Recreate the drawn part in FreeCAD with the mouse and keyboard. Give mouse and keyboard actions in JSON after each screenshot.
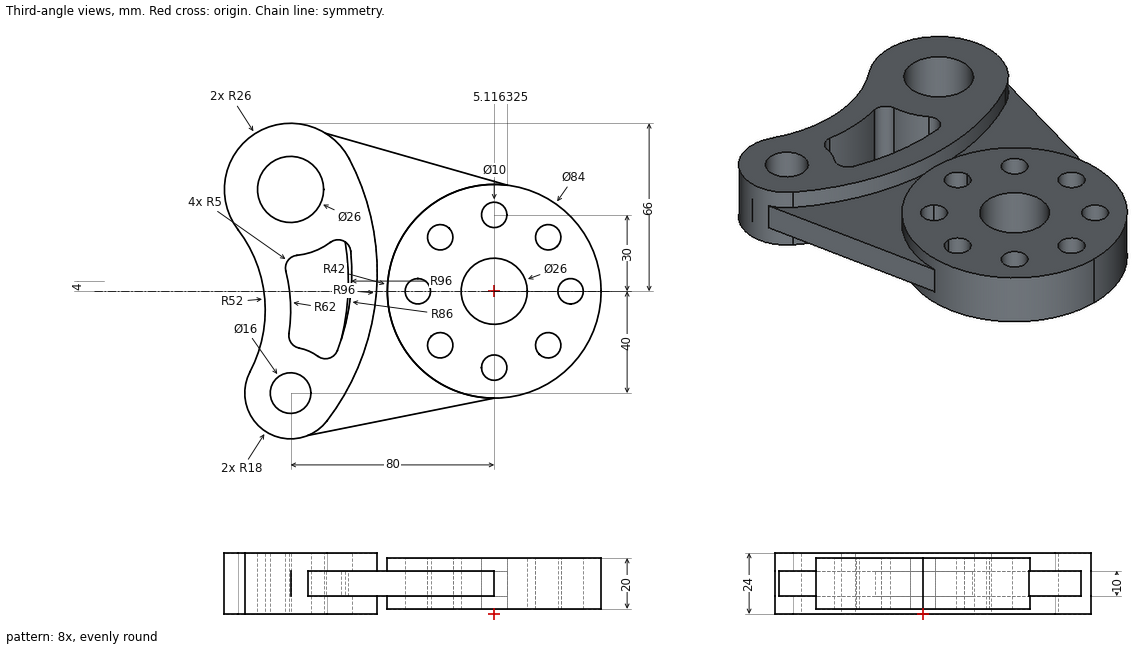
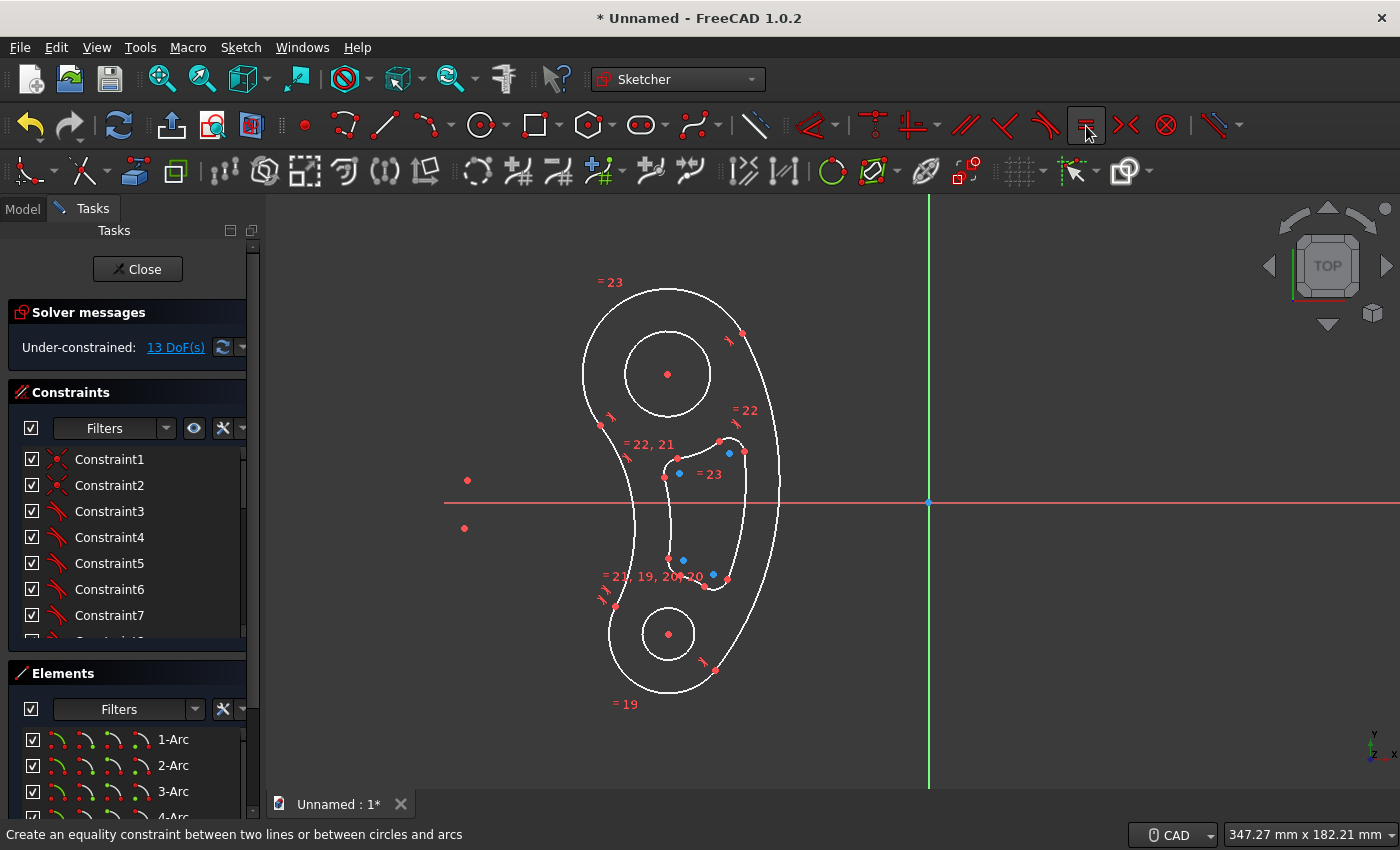
{"action": "left_click", "coordinate": [668, 374]}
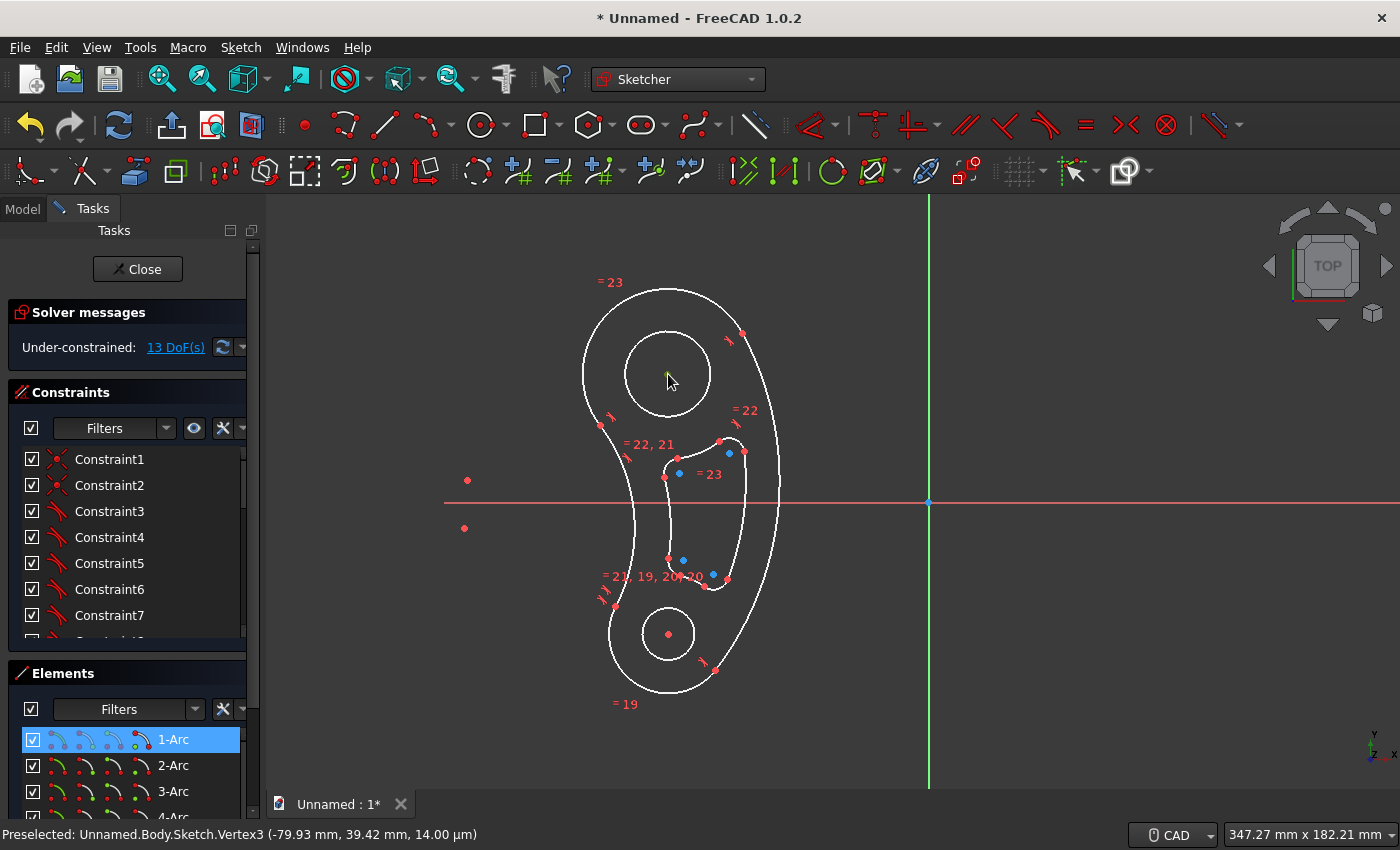
{"action": "left_click", "coordinate": [668, 634]}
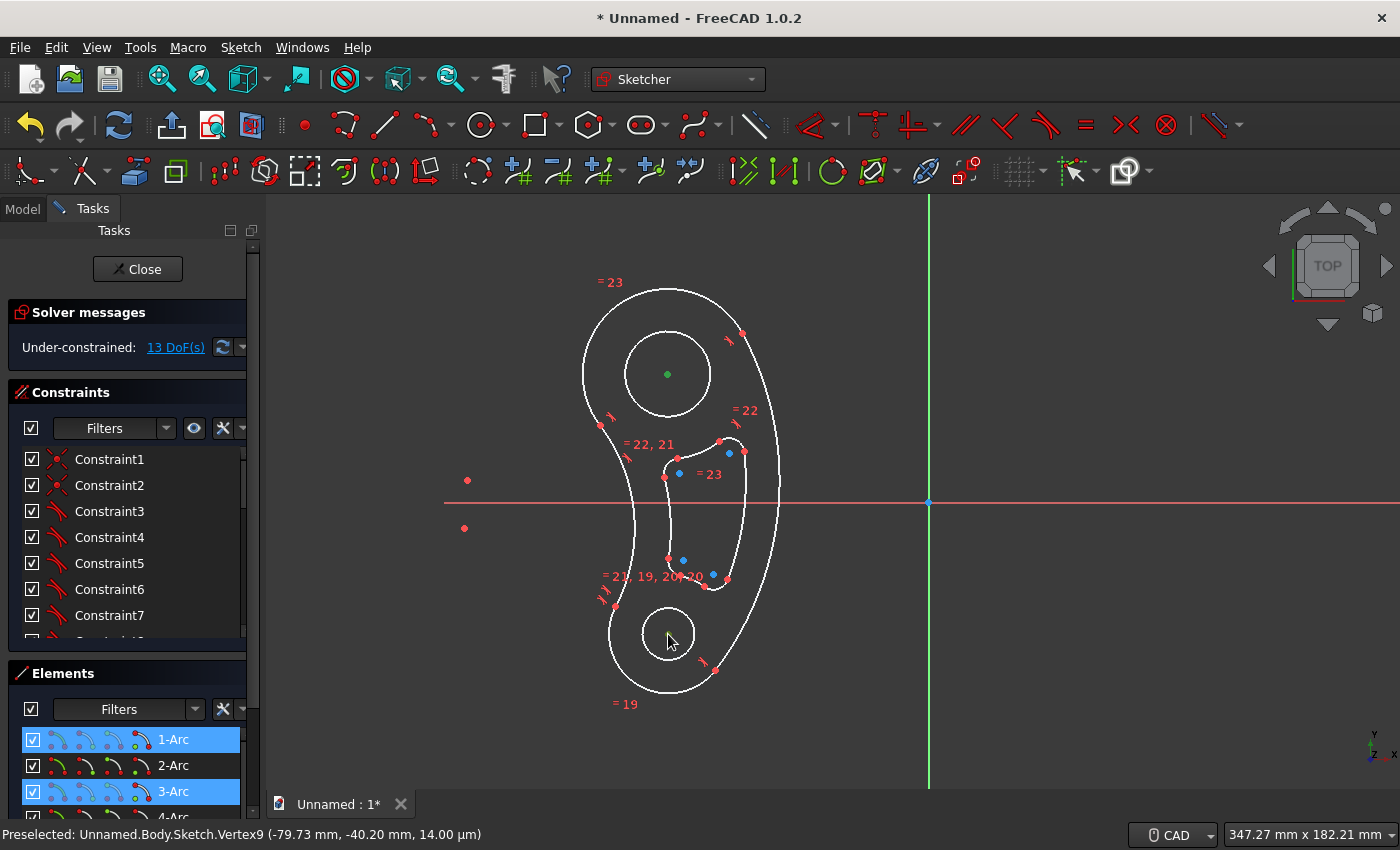
{"action": "left_click", "coordinate": [496, 503]}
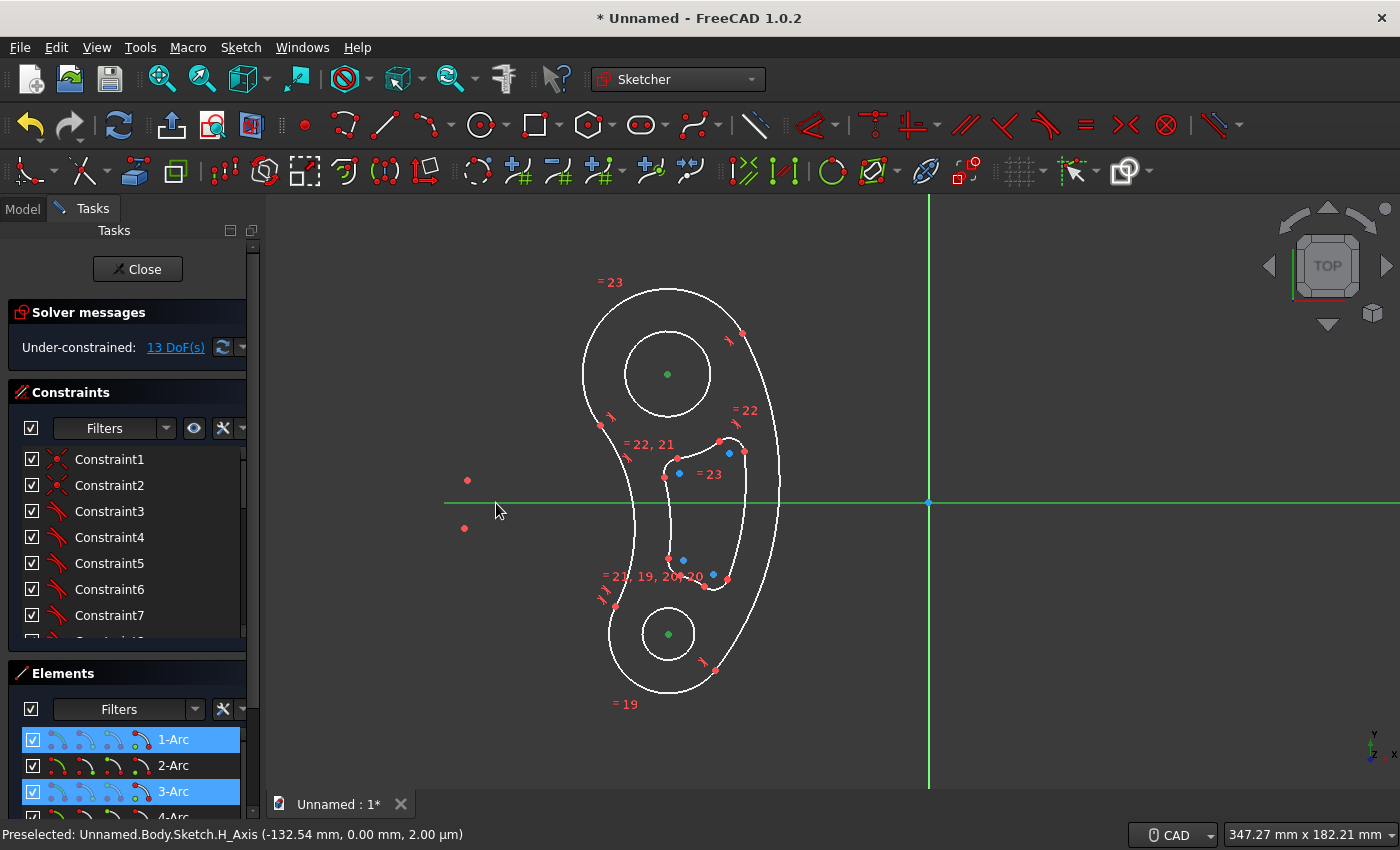
{"action": "left_click", "coordinate": [1126, 126]}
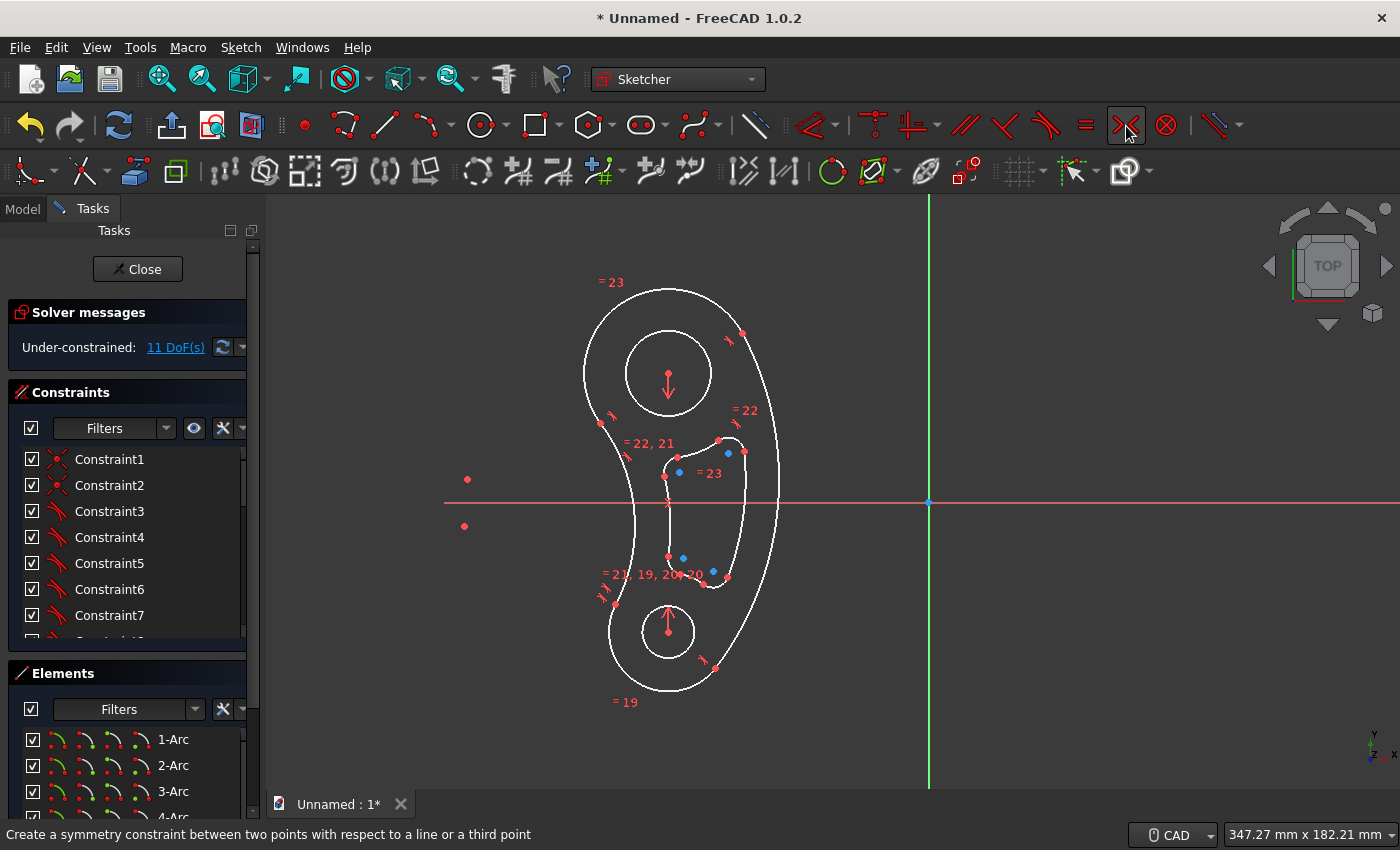
{"action": "left_click", "coordinate": [676, 290]}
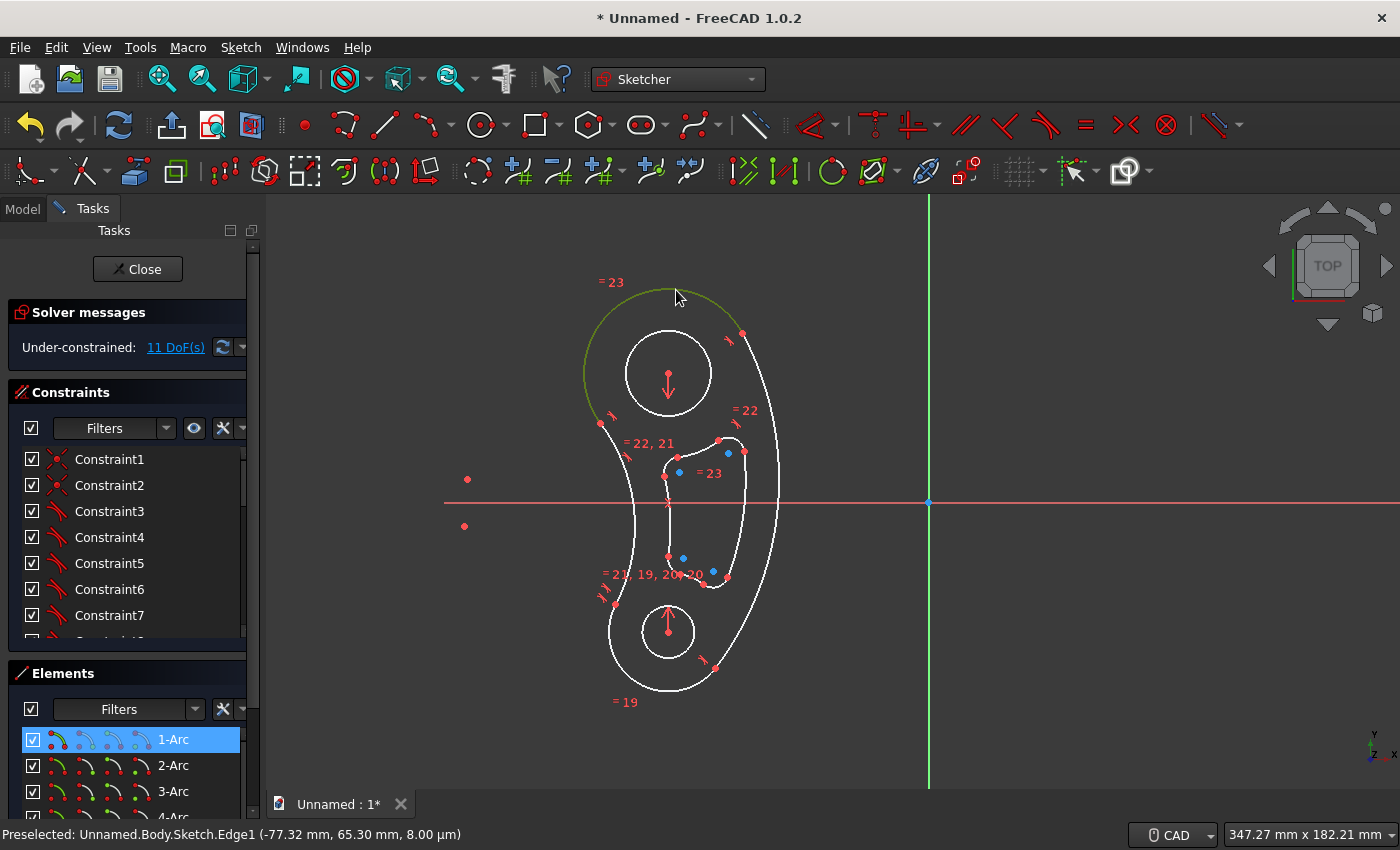
{"action": "left_click", "coordinate": [838, 126]}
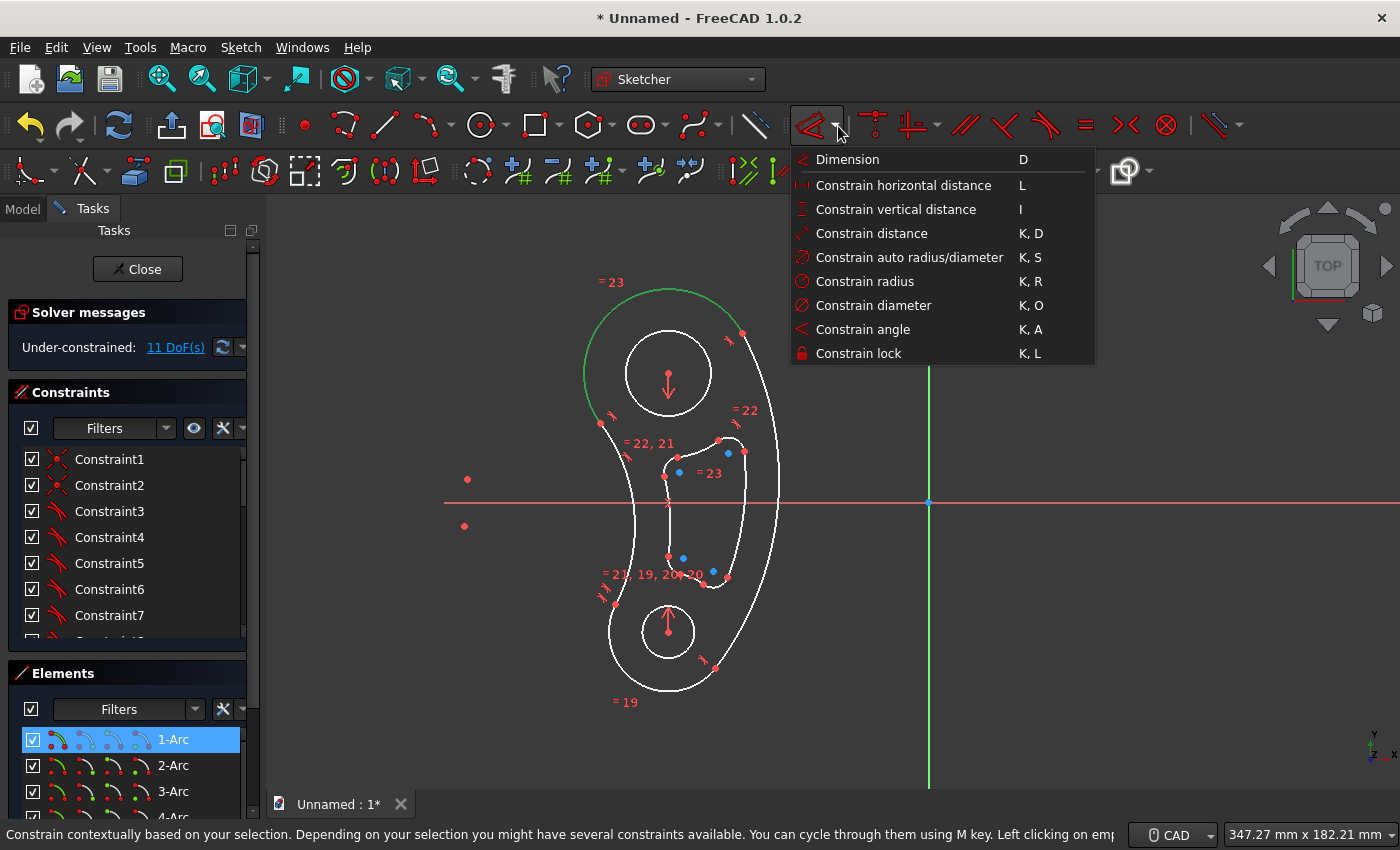
{"action": "left_click", "coordinate": [943, 281]}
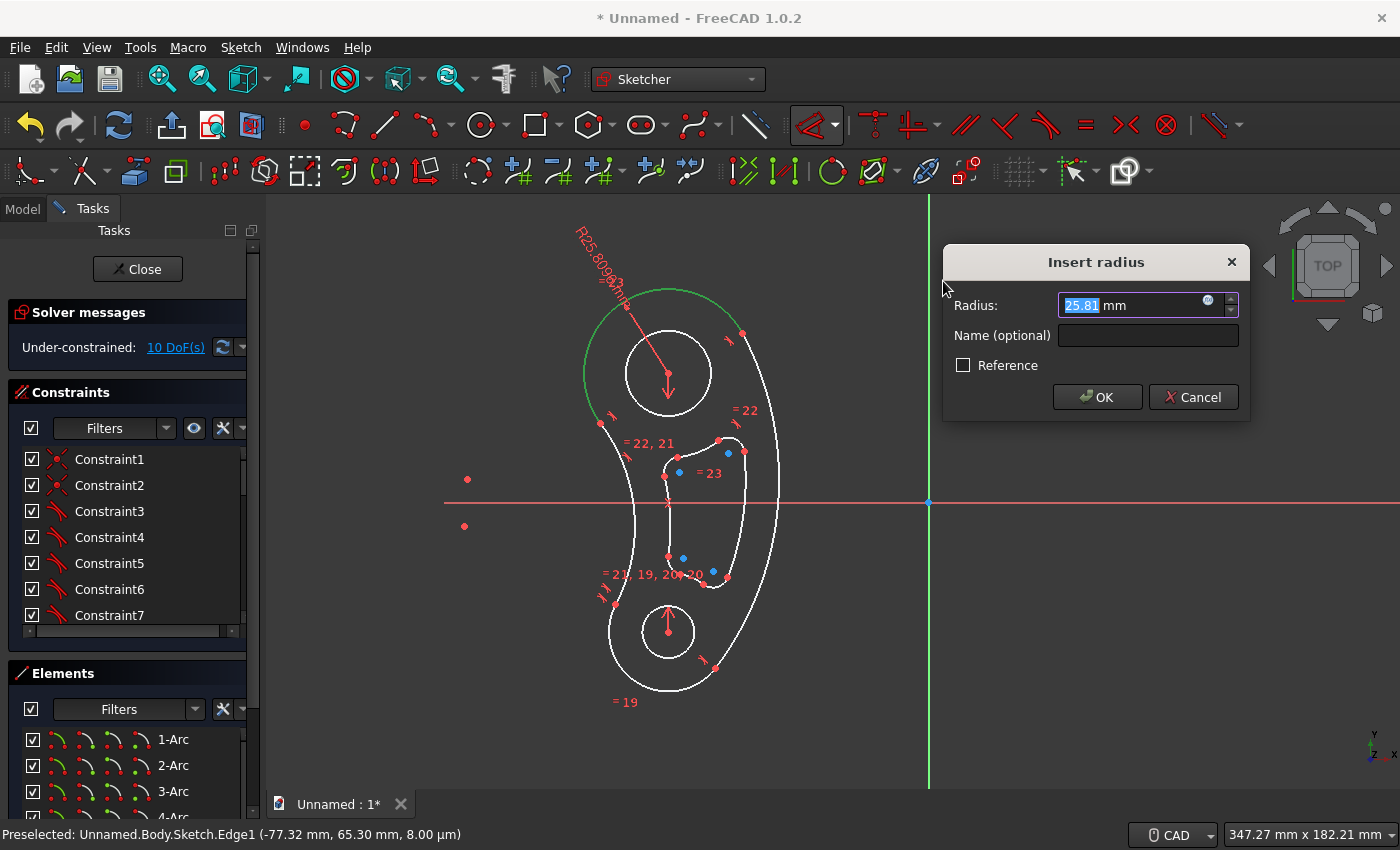
{"action": "type", "text": "26"}
{"action": "key", "text": "Return"}